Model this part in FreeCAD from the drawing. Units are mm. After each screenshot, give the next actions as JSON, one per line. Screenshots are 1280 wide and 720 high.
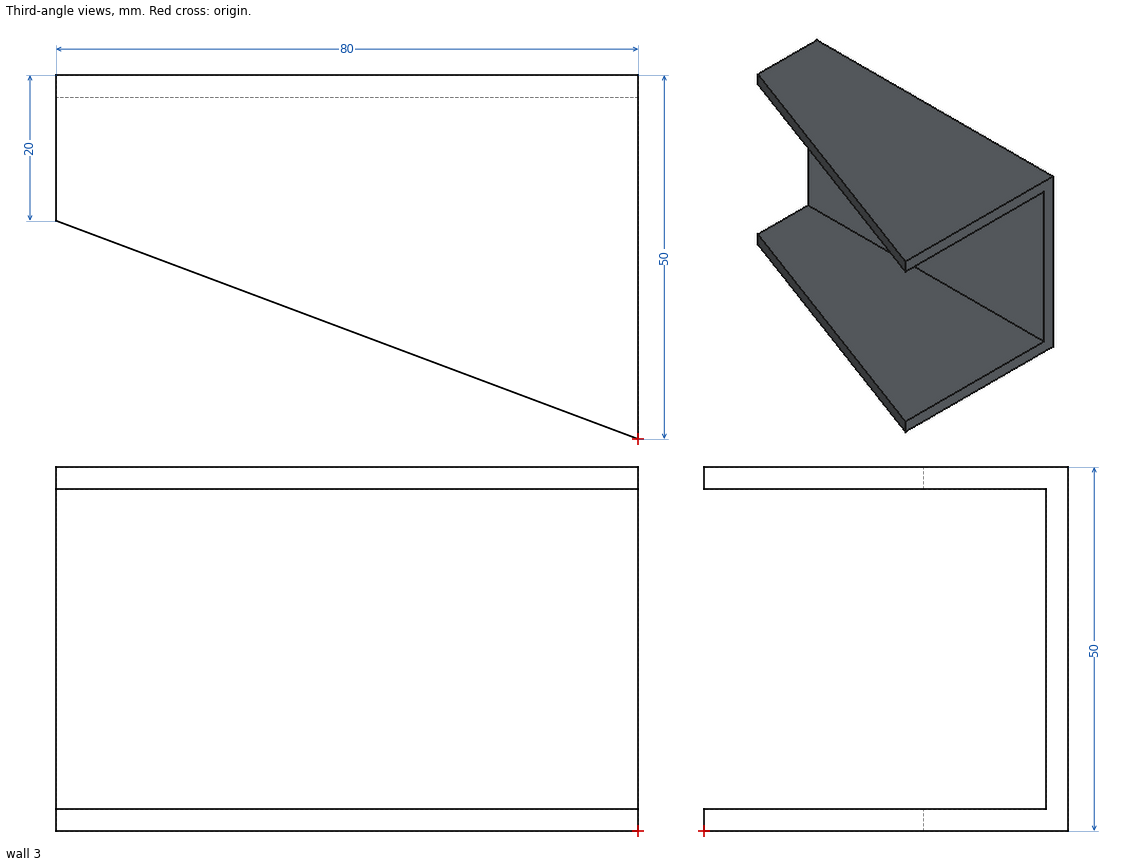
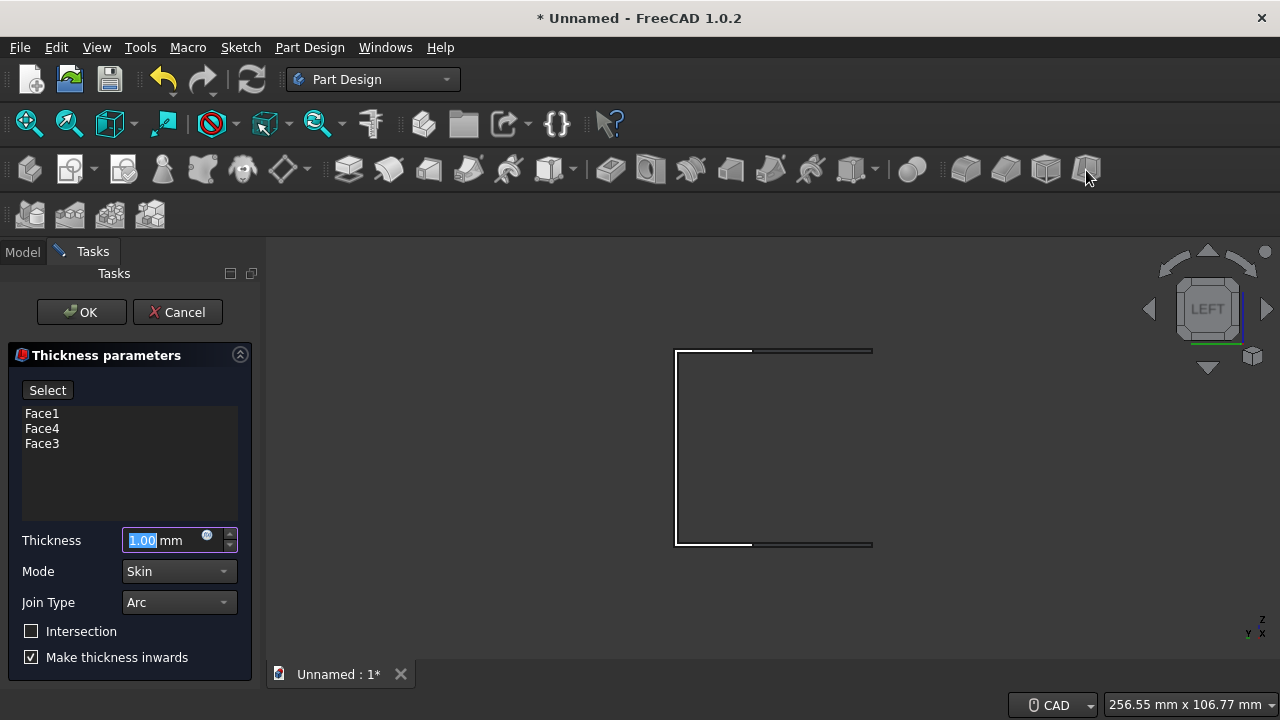
{"action": "type", "text": "3"}
{"action": "key", "text": "Tab"}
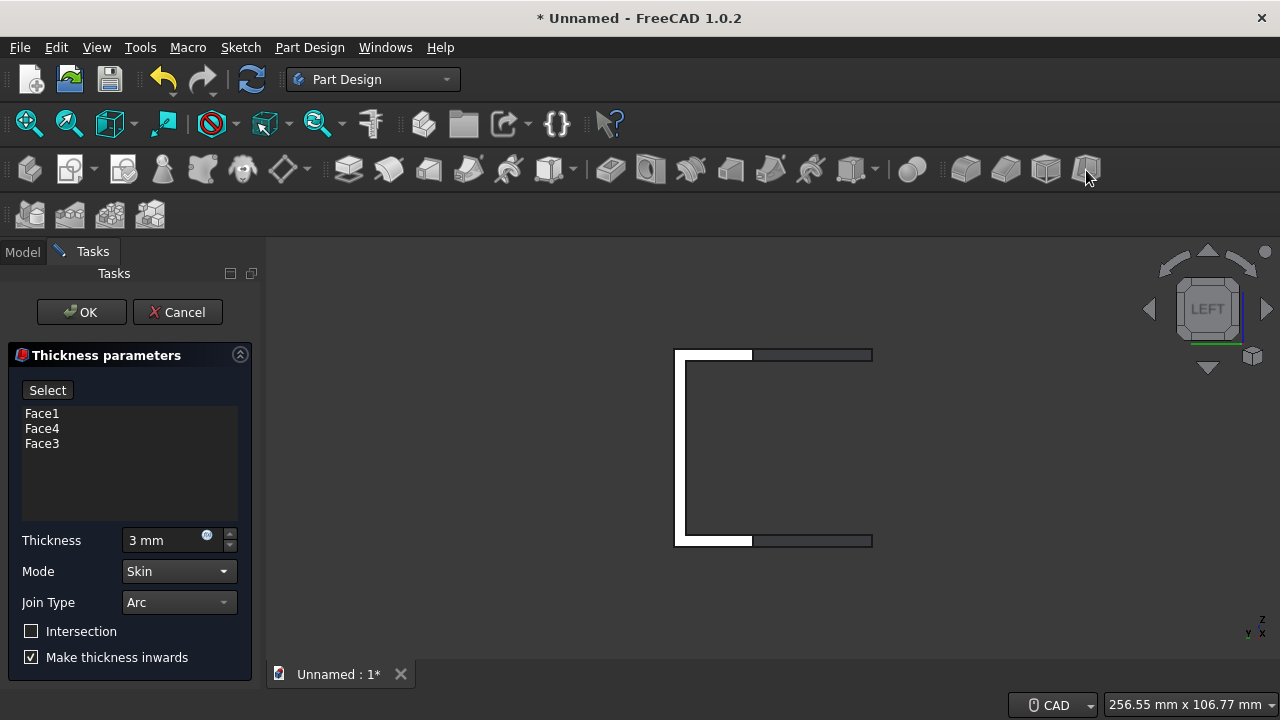
{"action": "left_click", "coordinate": [180, 602]}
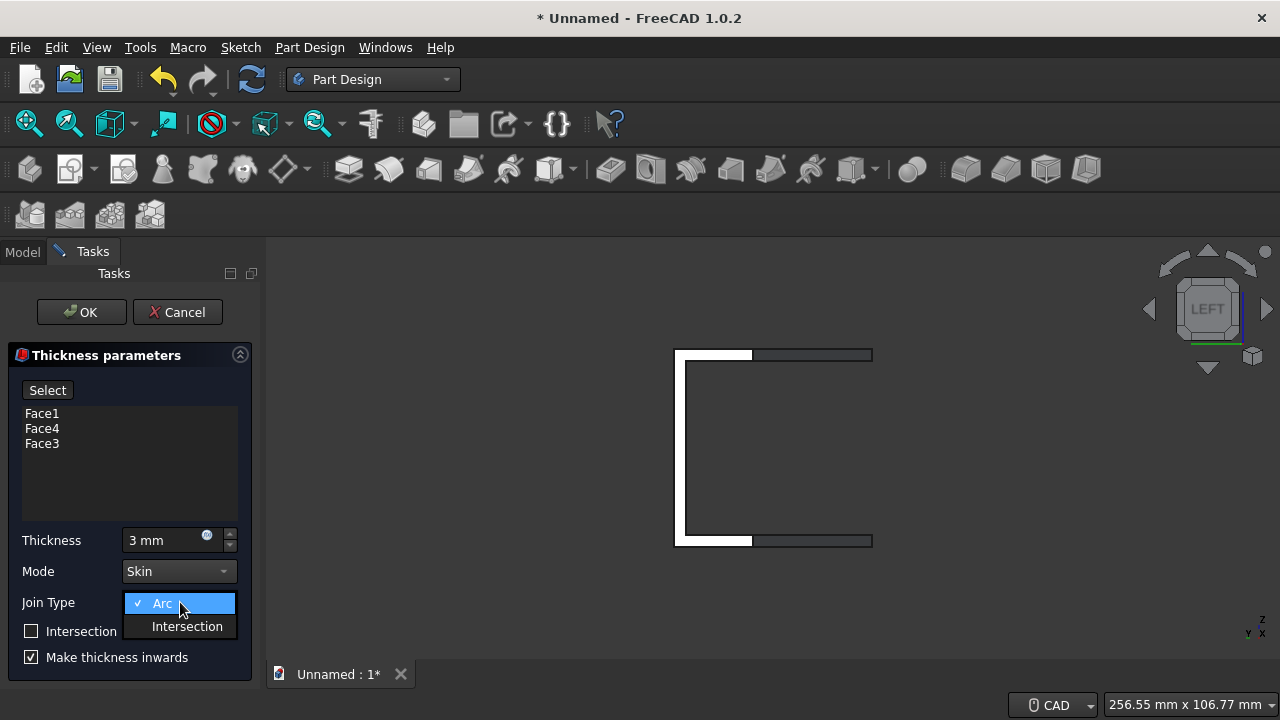
{"action": "left_click", "coordinate": [179, 626]}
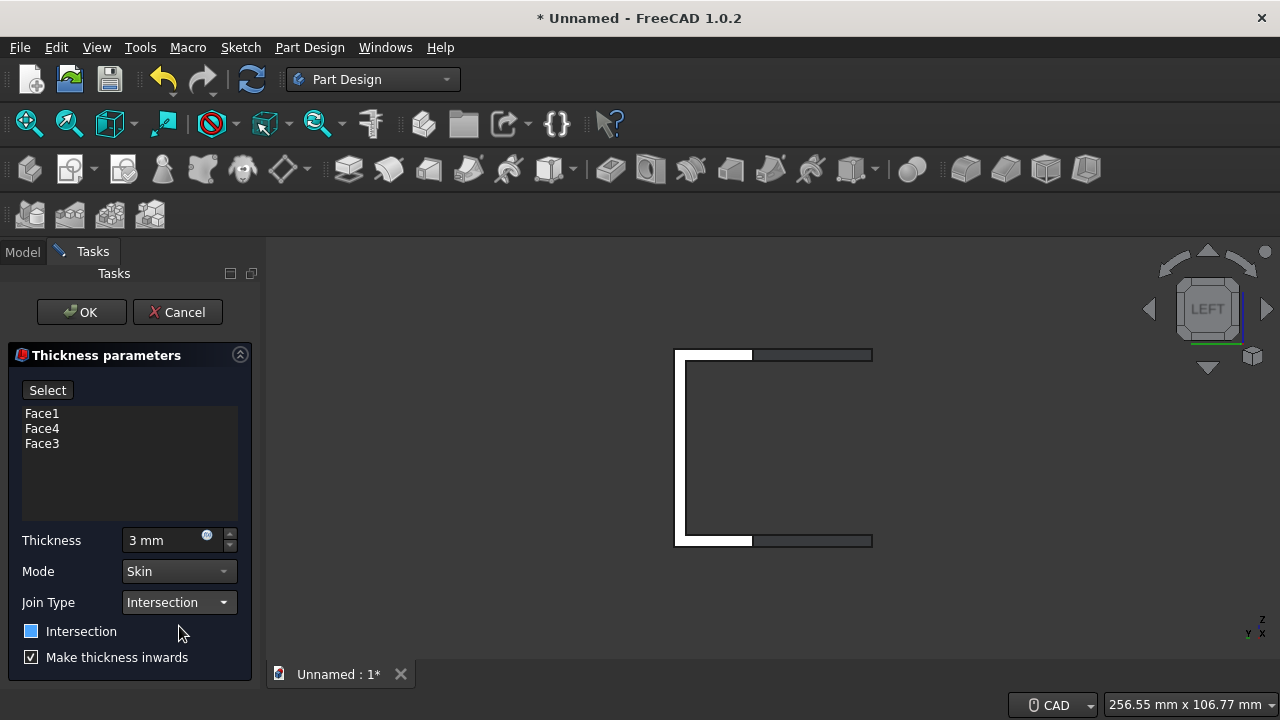
{"action": "left_click", "coordinate": [82, 312]}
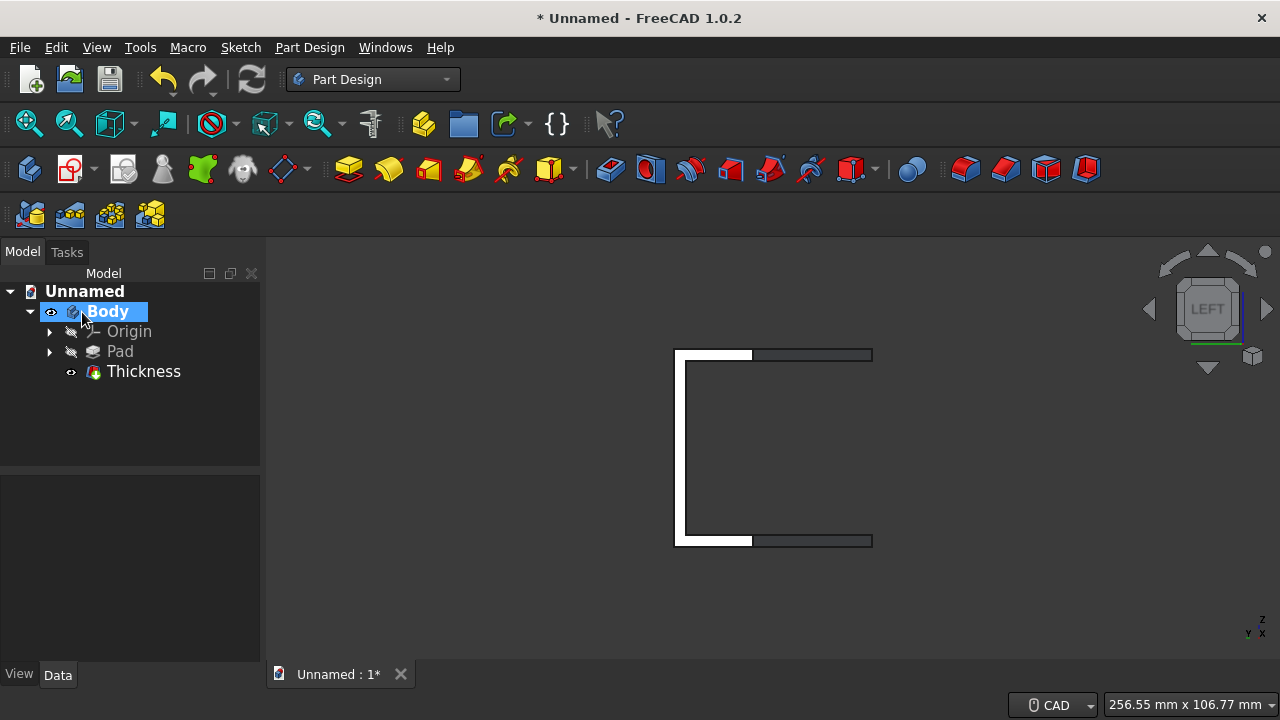
{"action": "key", "text": "0"}